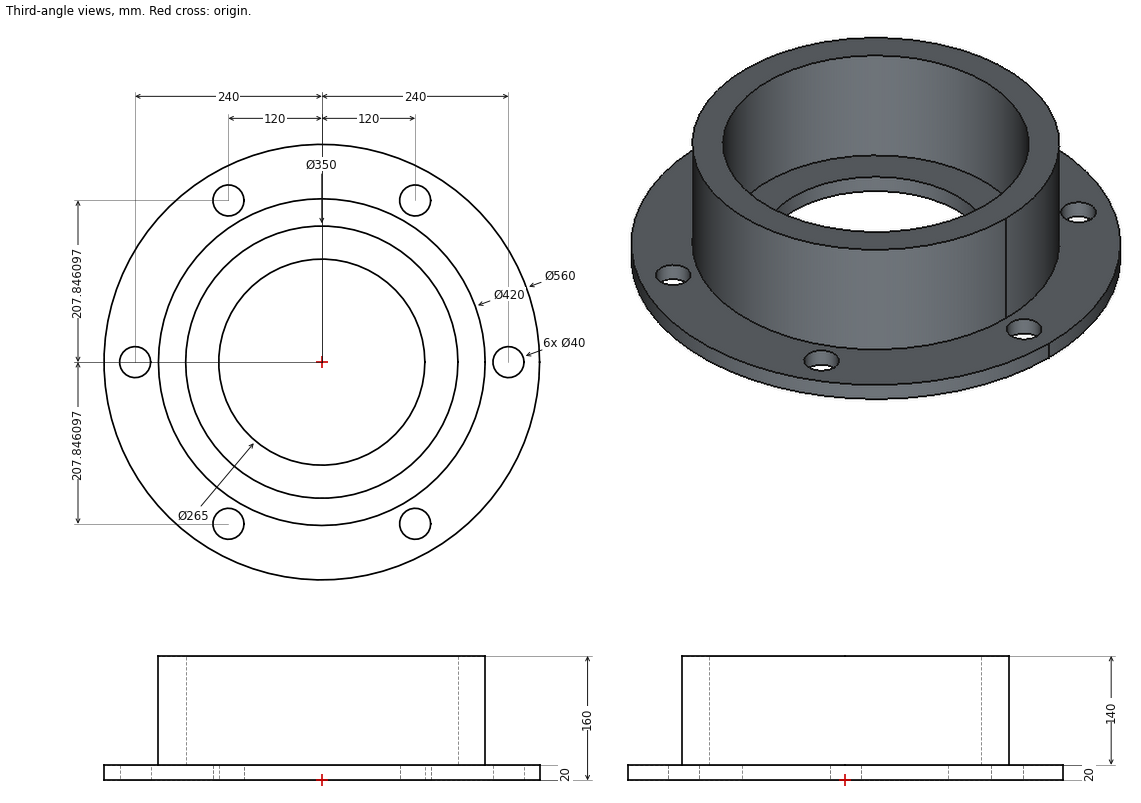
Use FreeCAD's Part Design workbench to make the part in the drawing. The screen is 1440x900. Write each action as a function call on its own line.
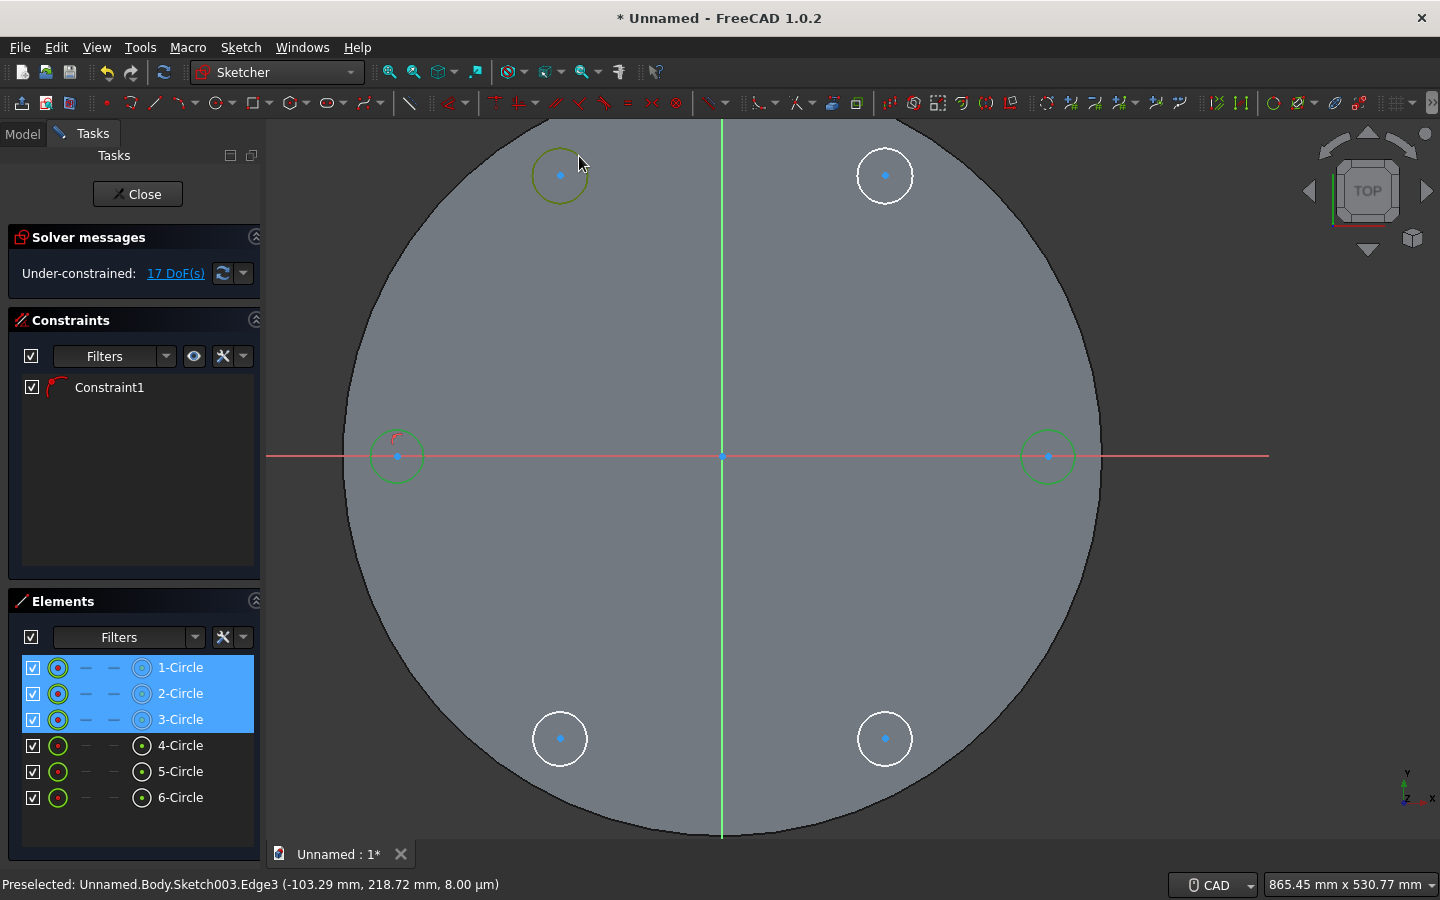
click(904, 156)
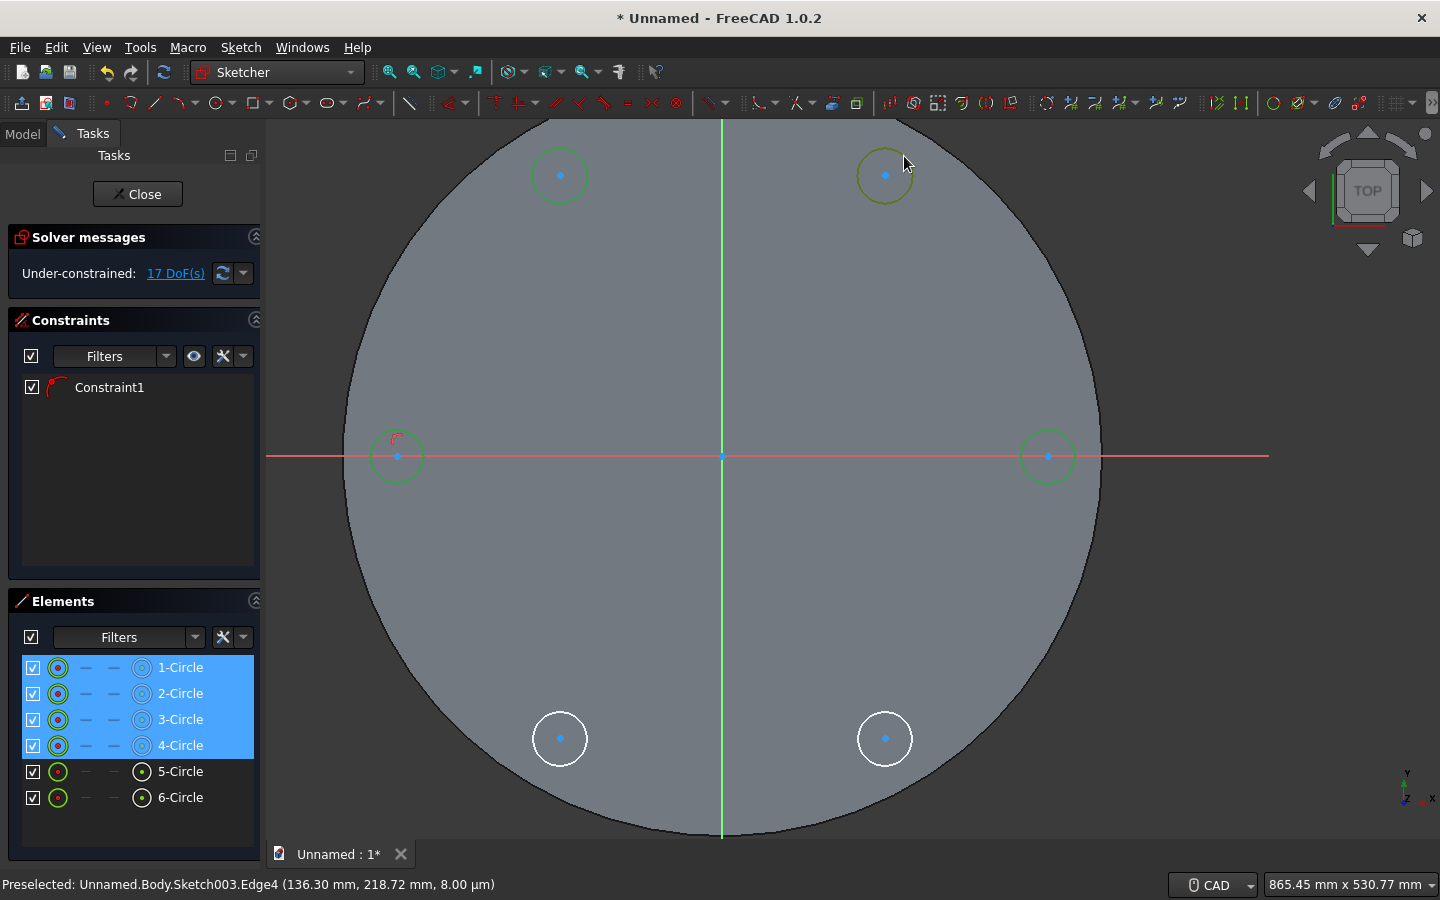
click(579, 720)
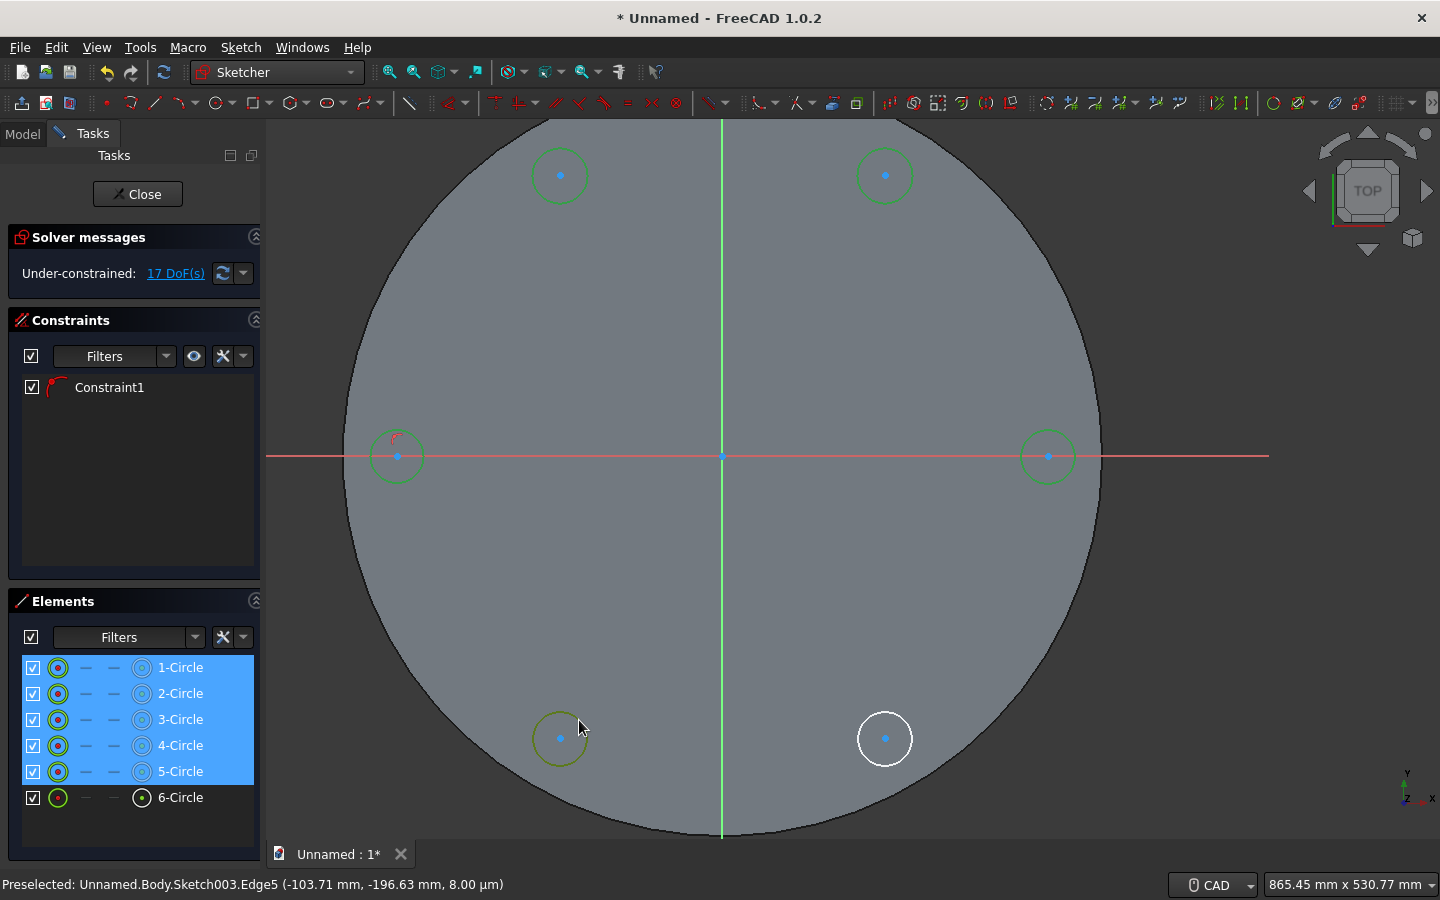
click(904, 720)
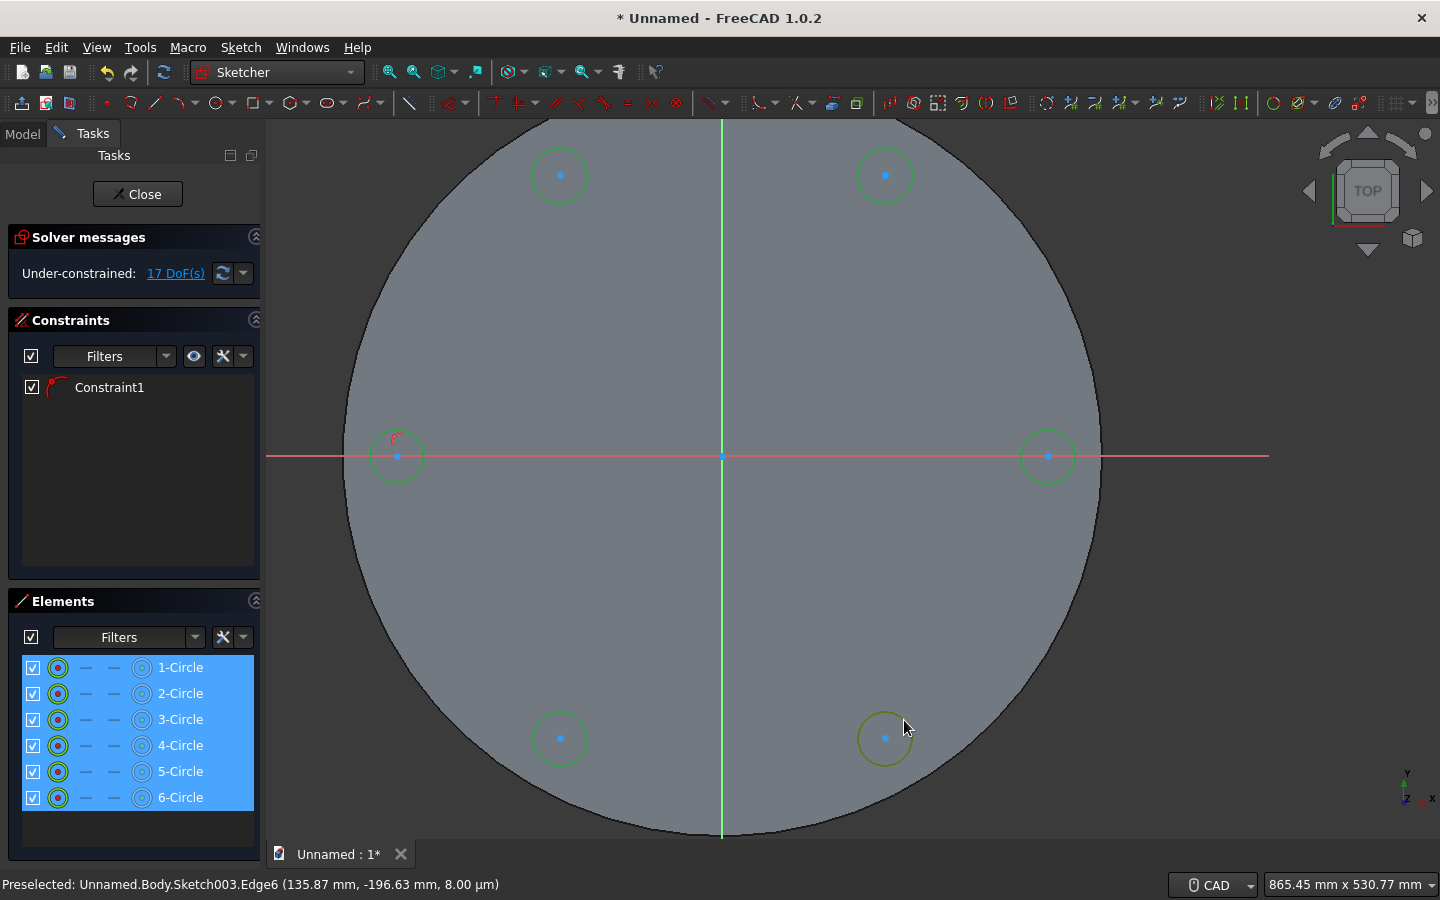
key(e)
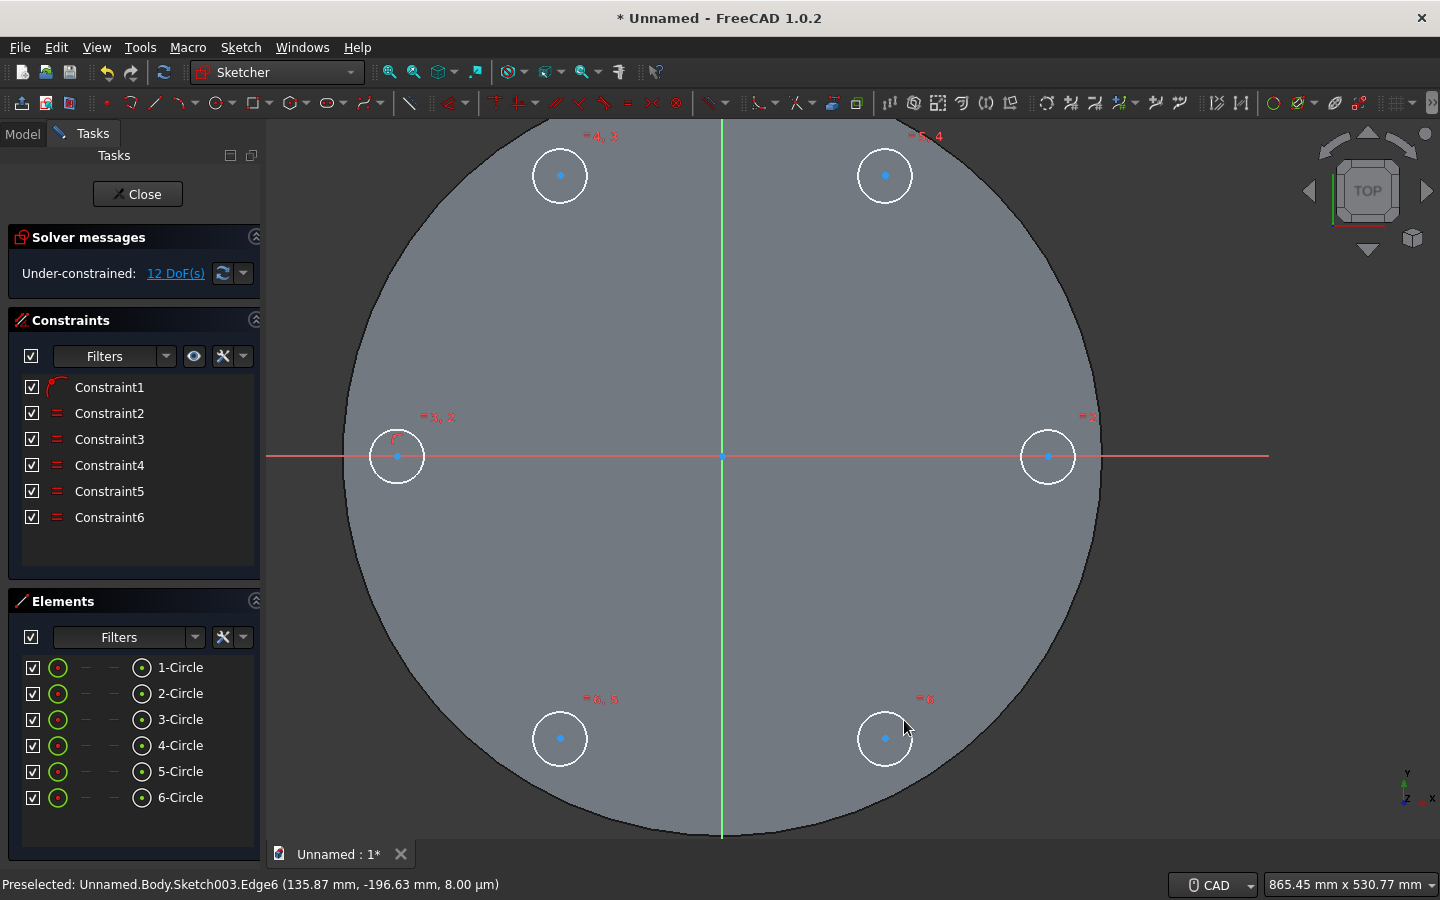
click(1048, 457)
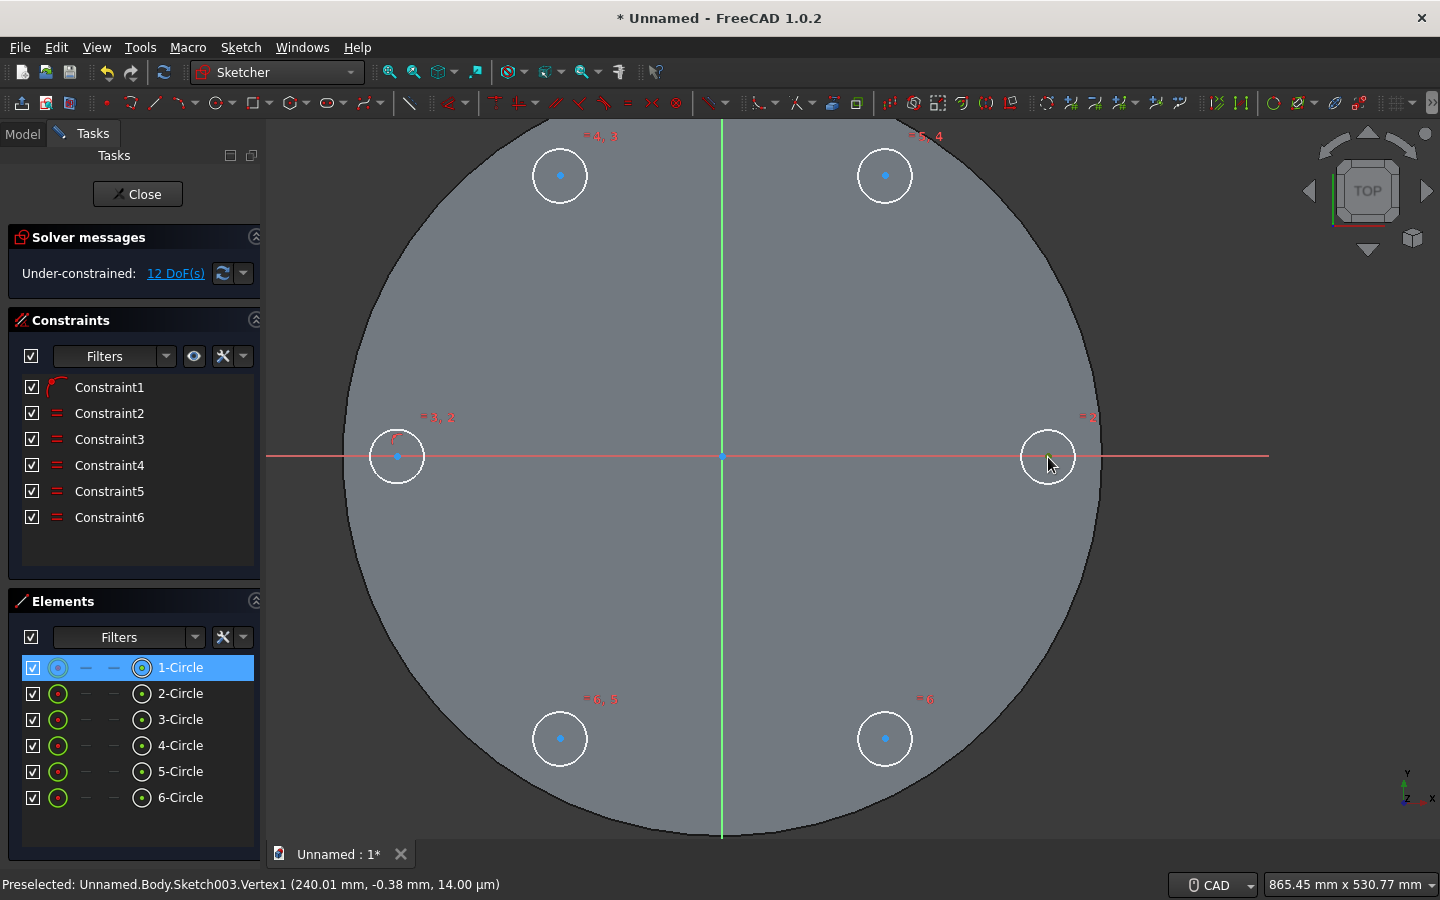
click(504, 456)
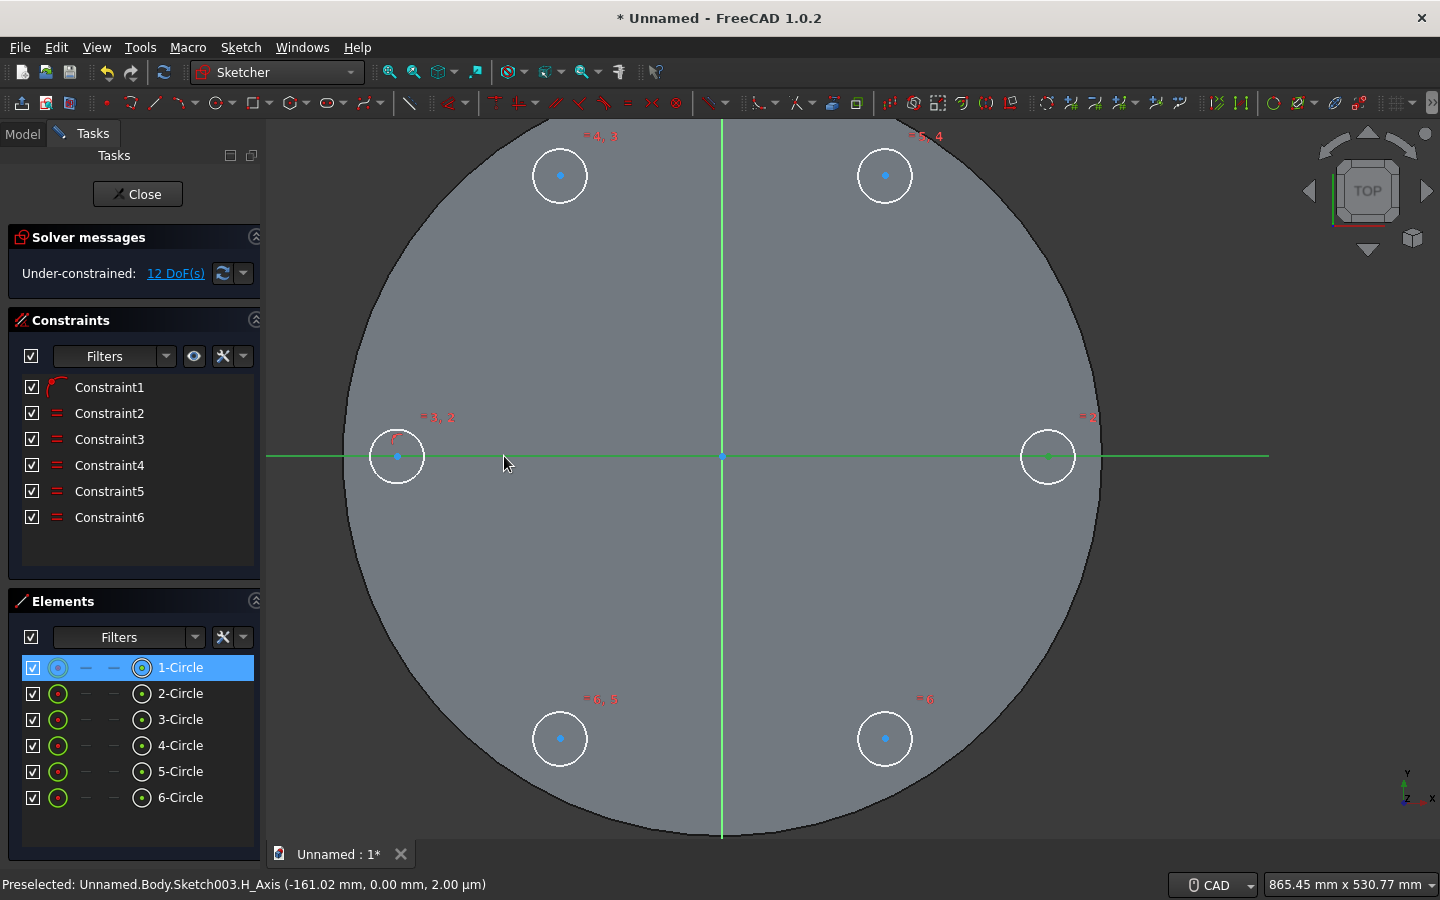
key(c)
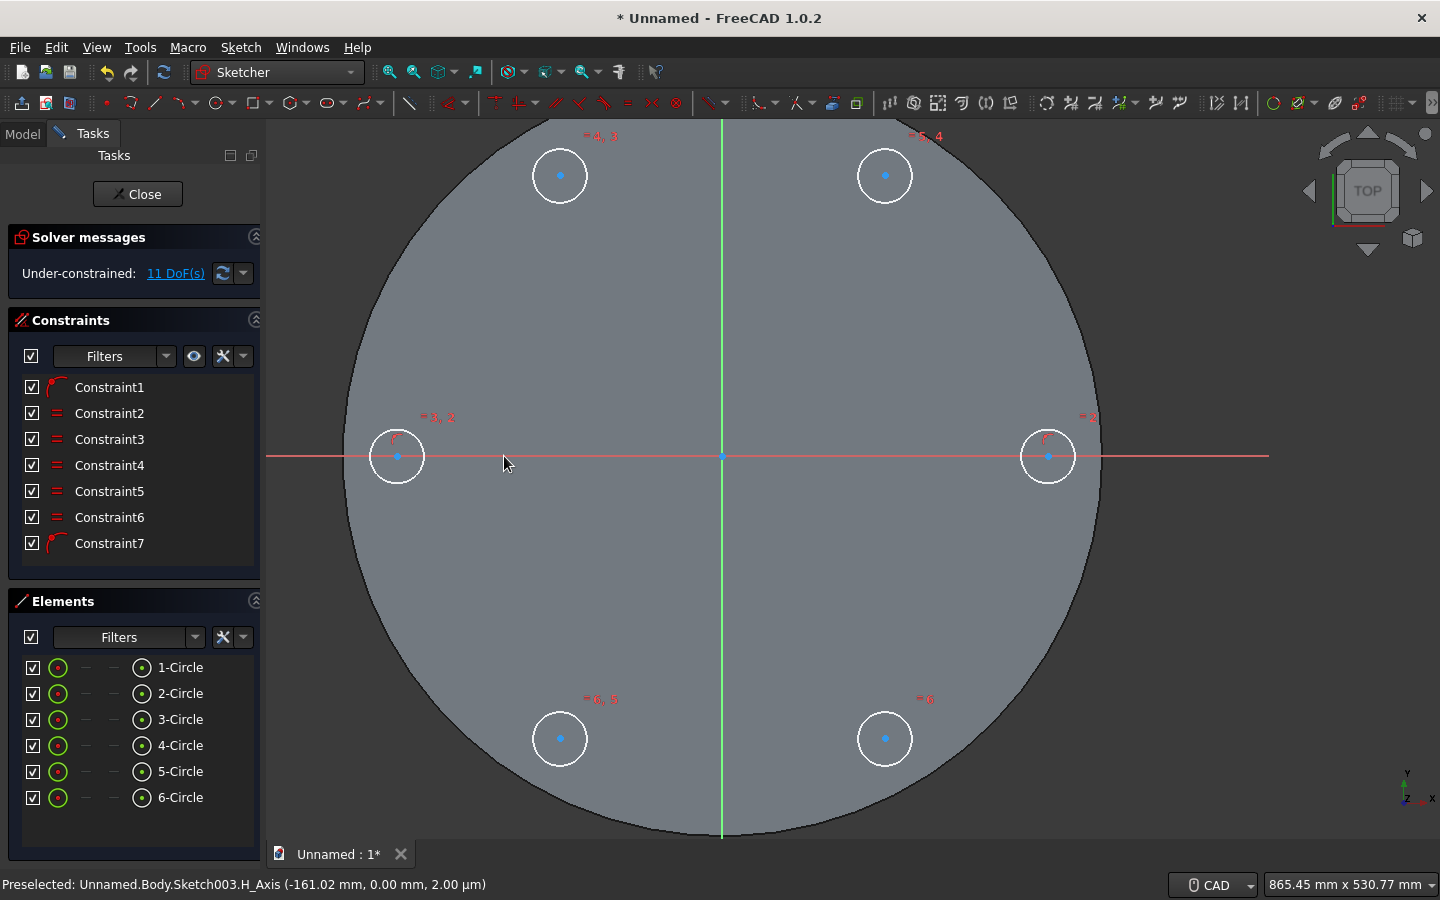
click(560, 176)